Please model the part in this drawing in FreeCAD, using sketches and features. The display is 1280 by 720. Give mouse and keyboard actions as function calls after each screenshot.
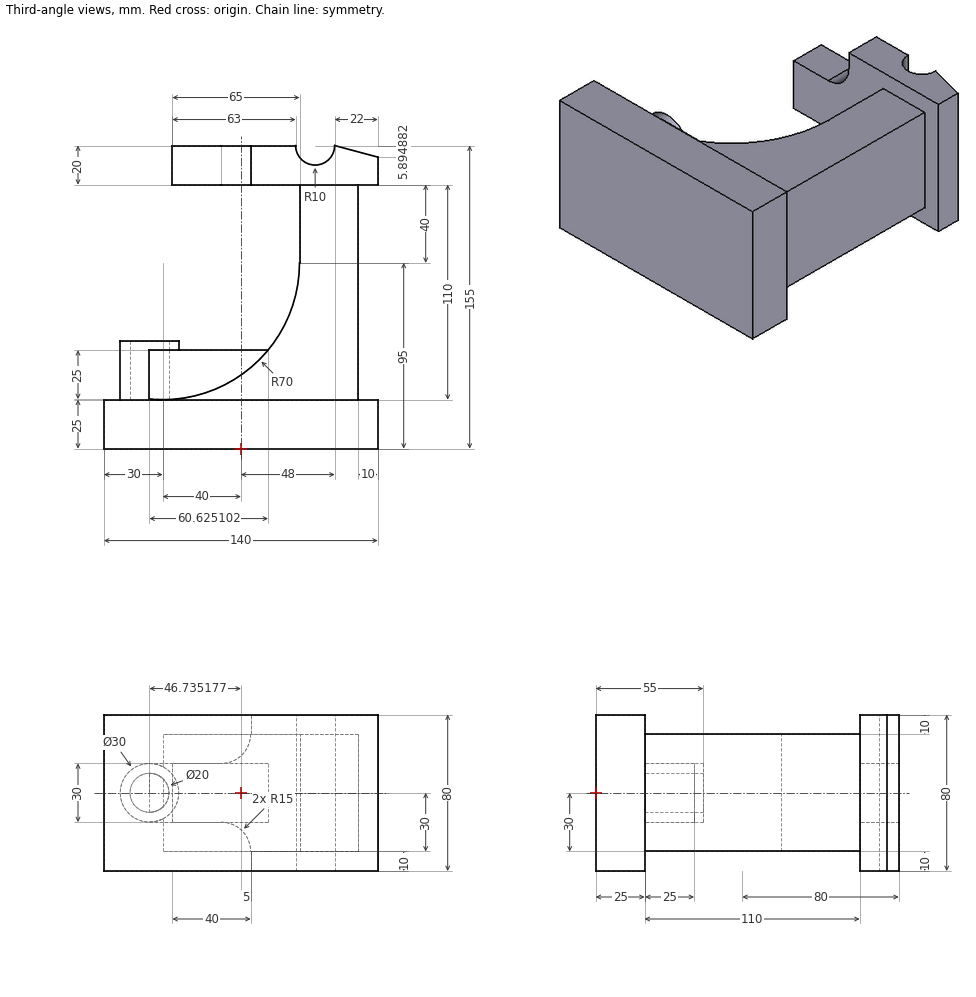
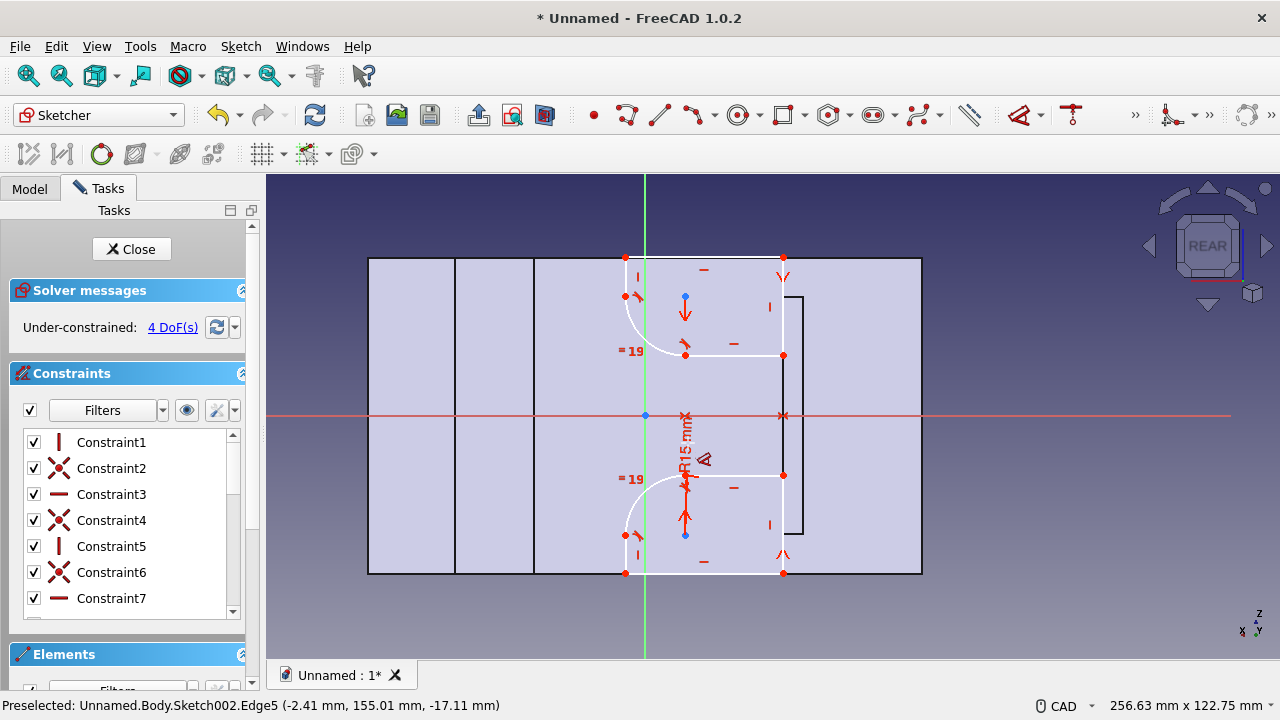
click(626, 547)
click(592, 554)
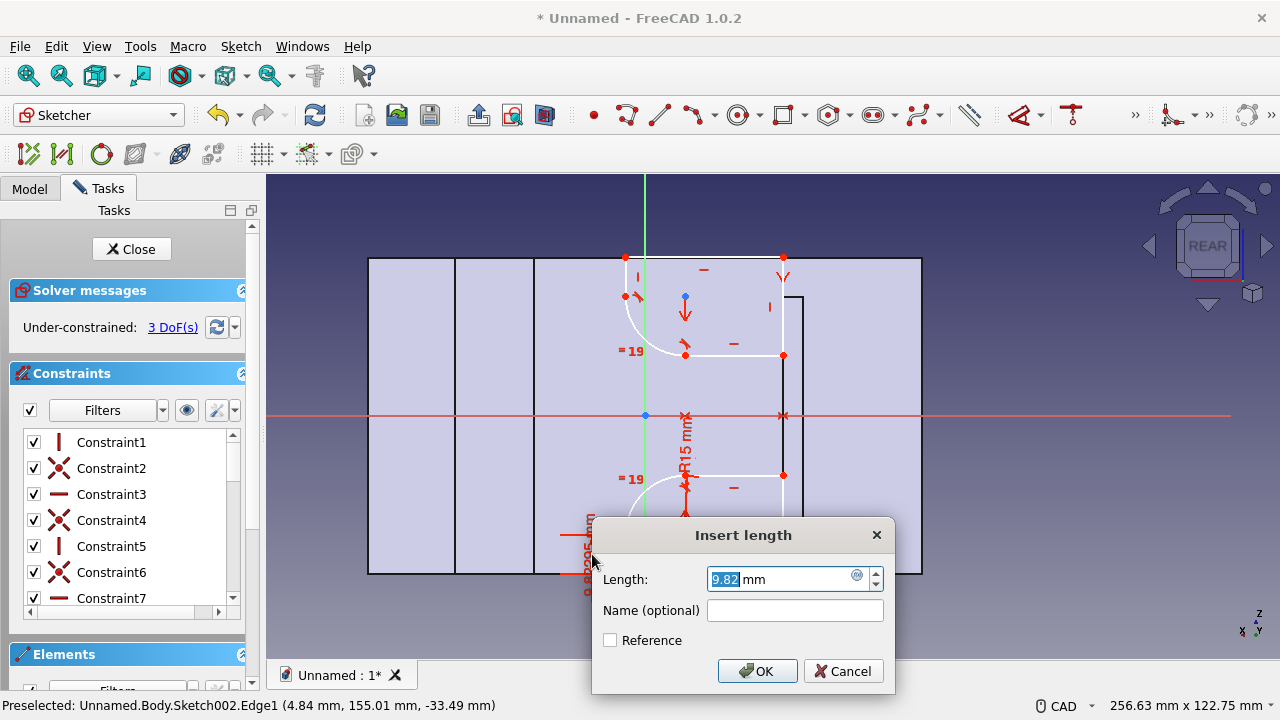
text(10)
key(Return)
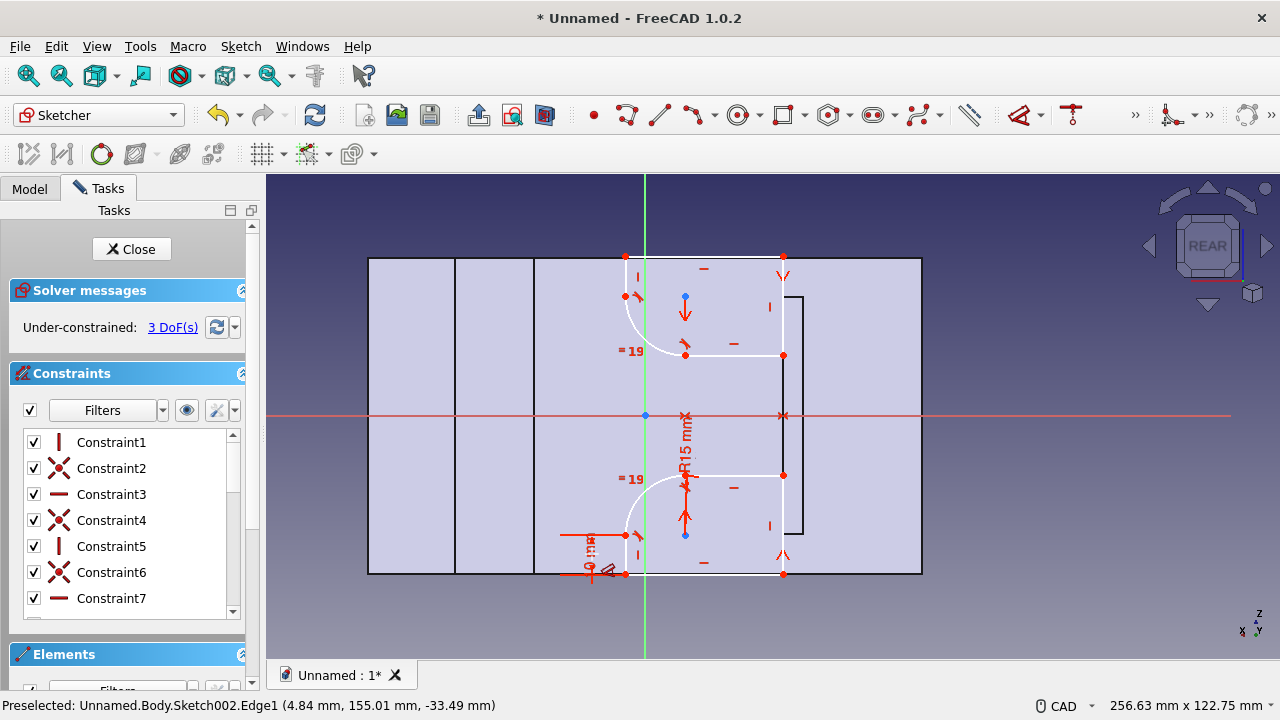
click(673, 575)
click(704, 609)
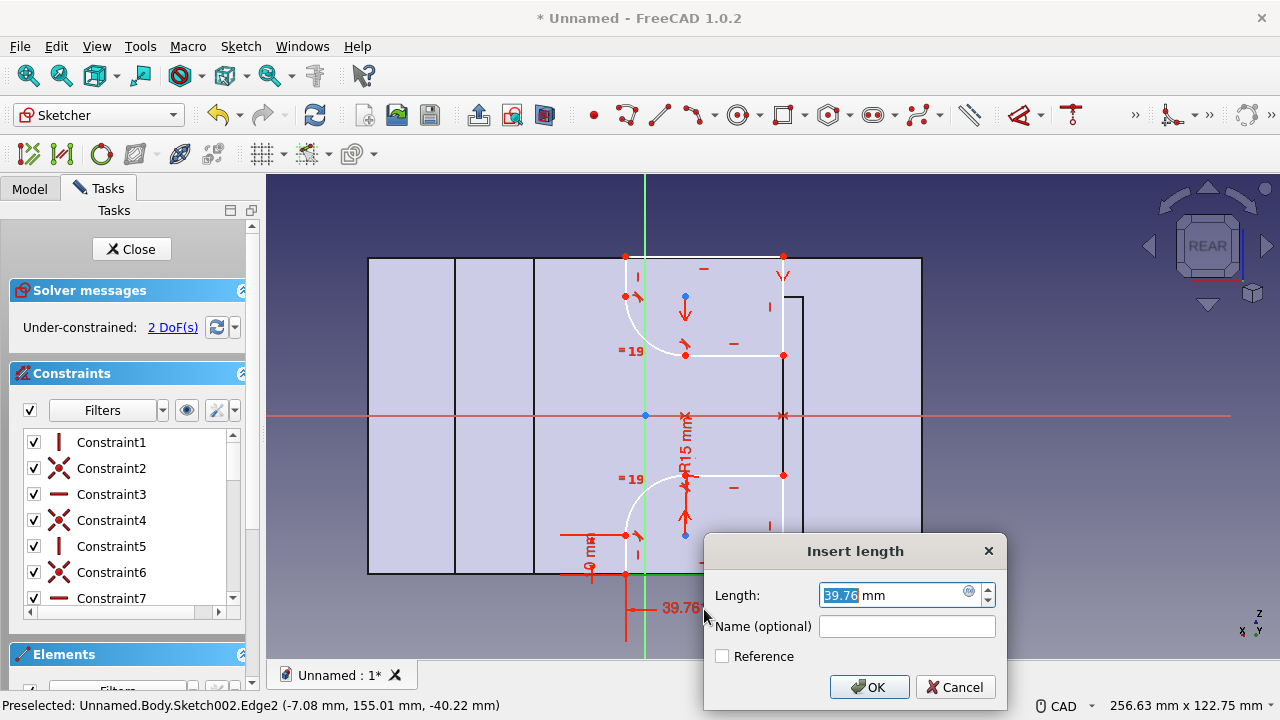
text(40)
key(Return)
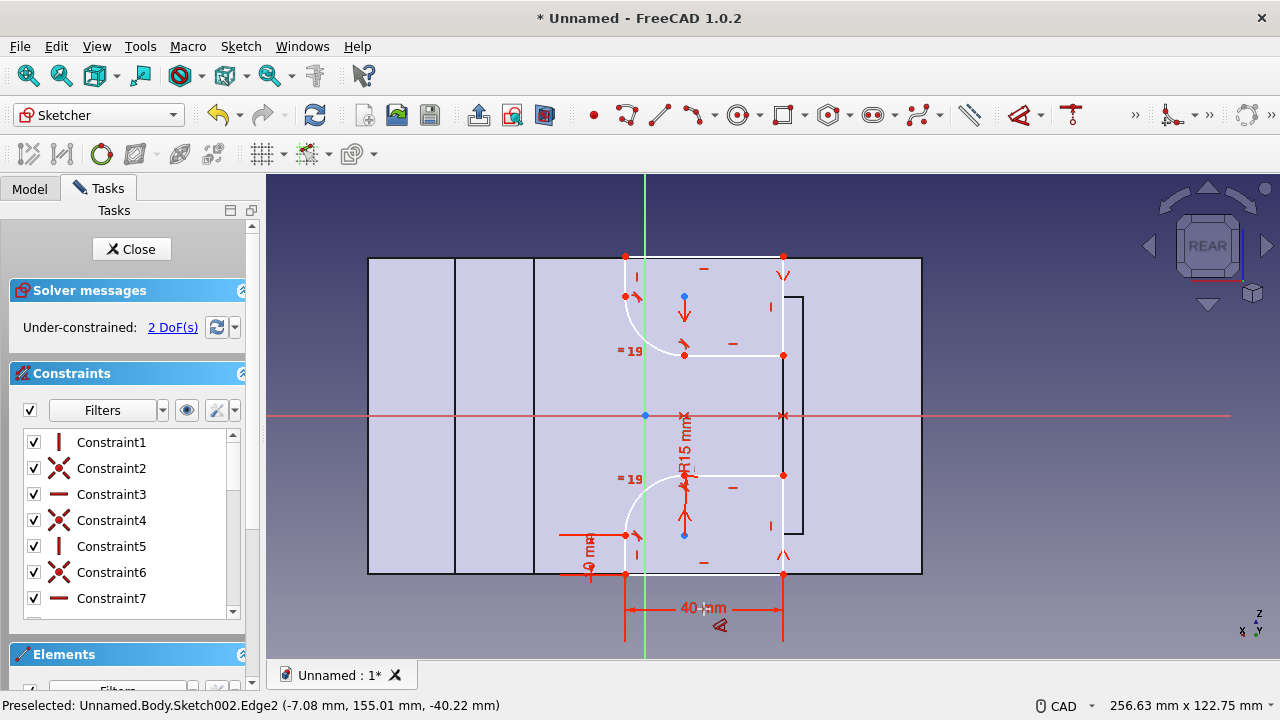
scroll(625, 535, up, 4)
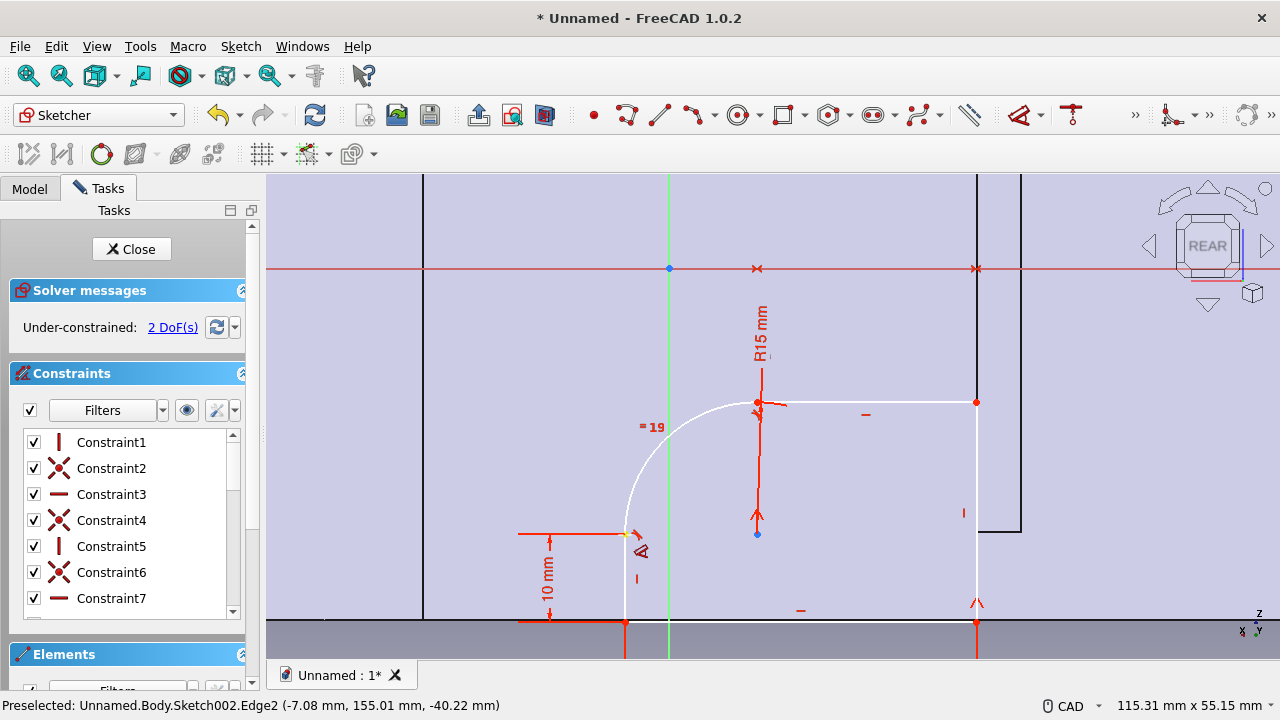
click(625, 534)
click(647, 568)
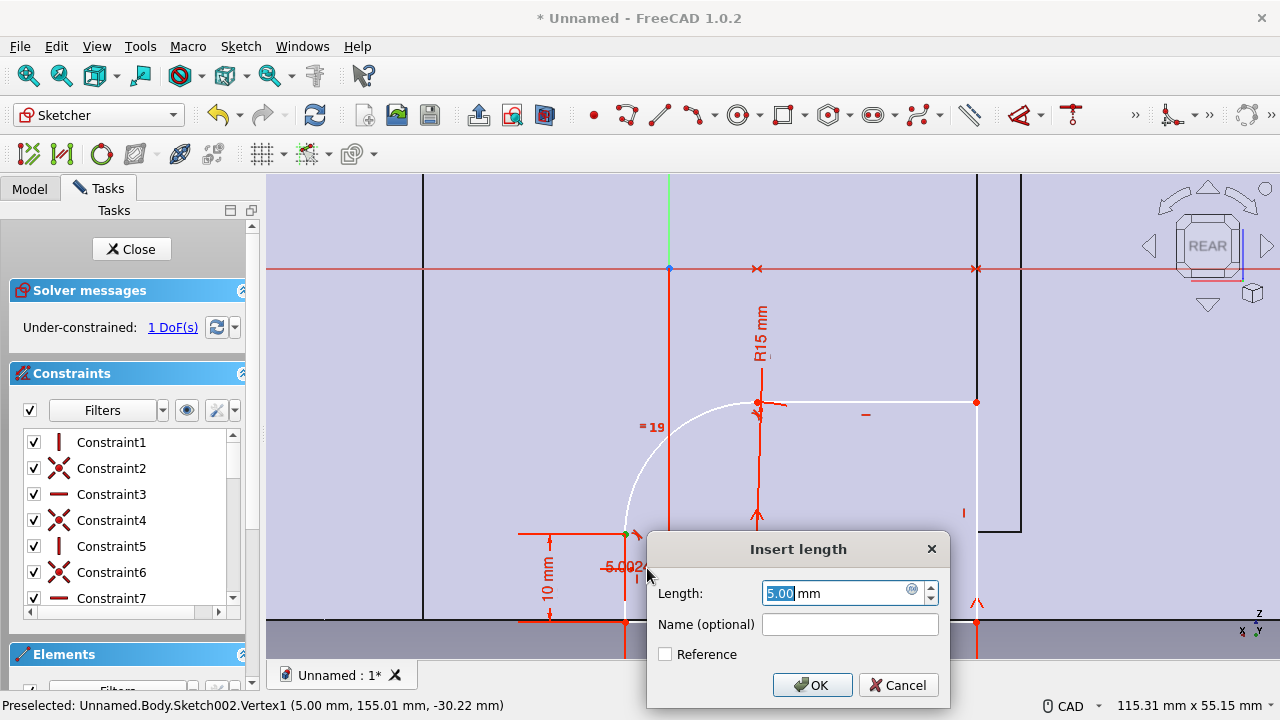
text(5)
key(Return)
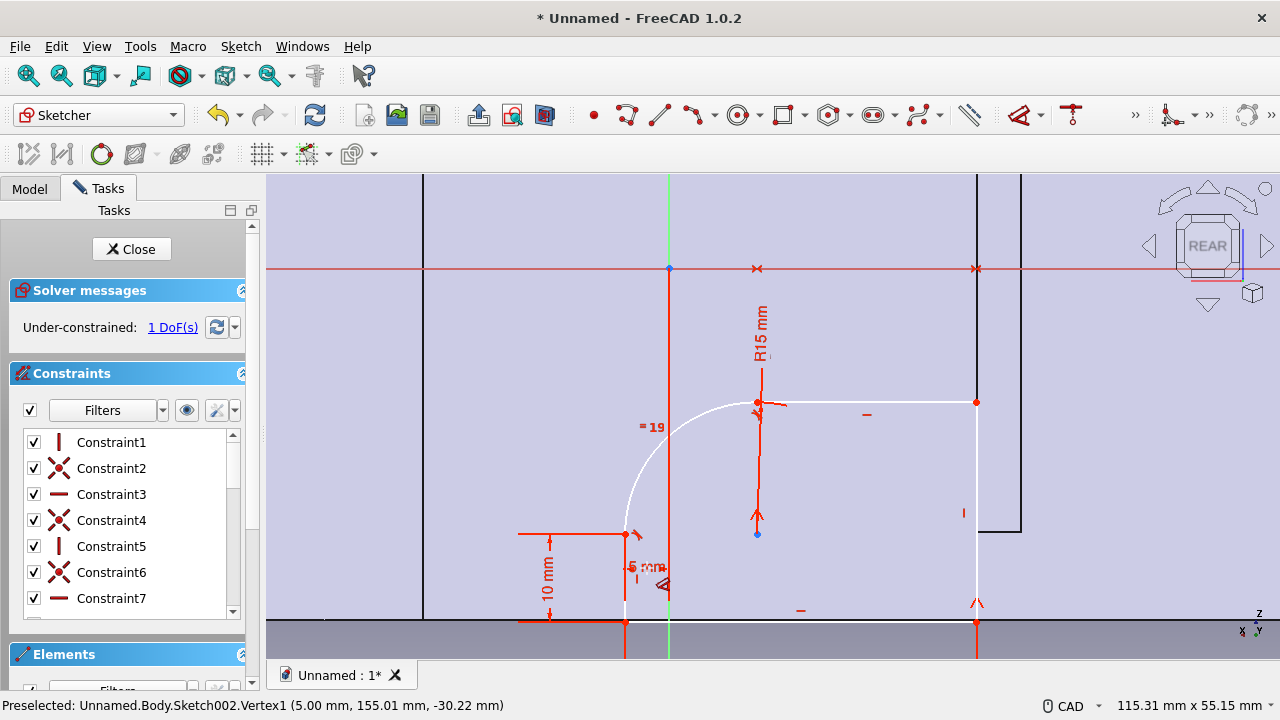
click(625, 534)
click(591, 401)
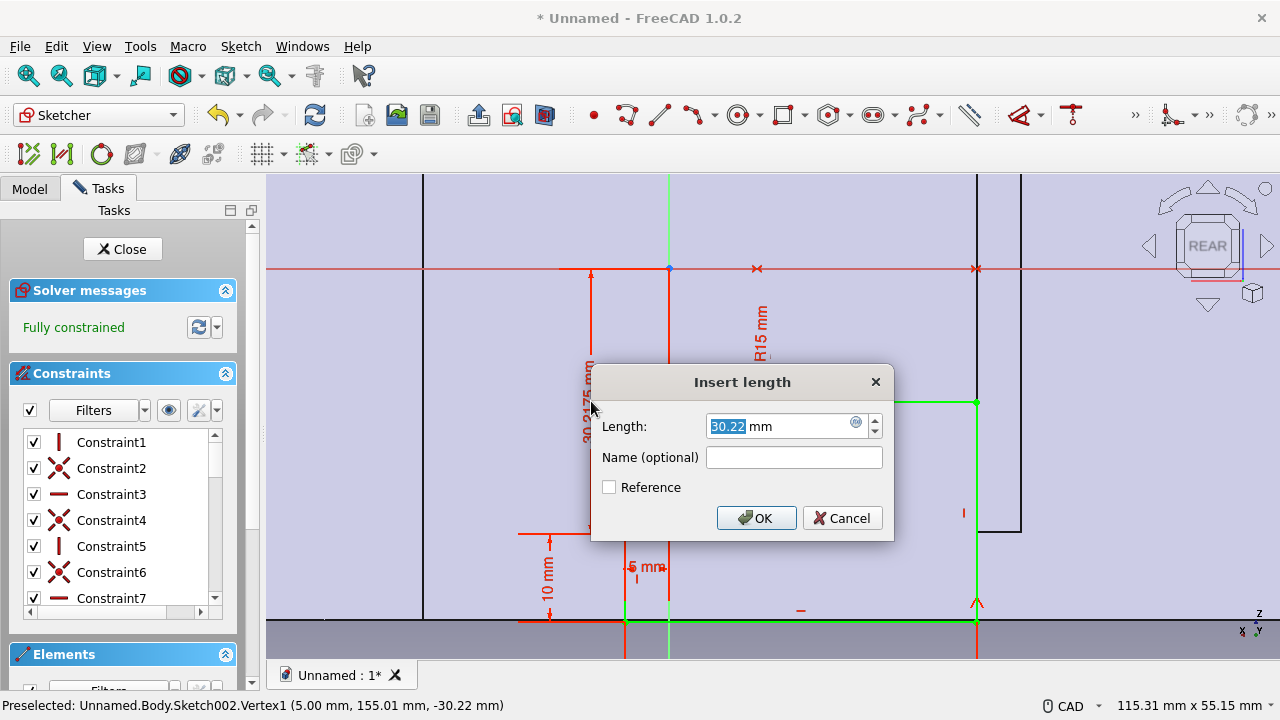
text(30)
key(Return)
key(Escape)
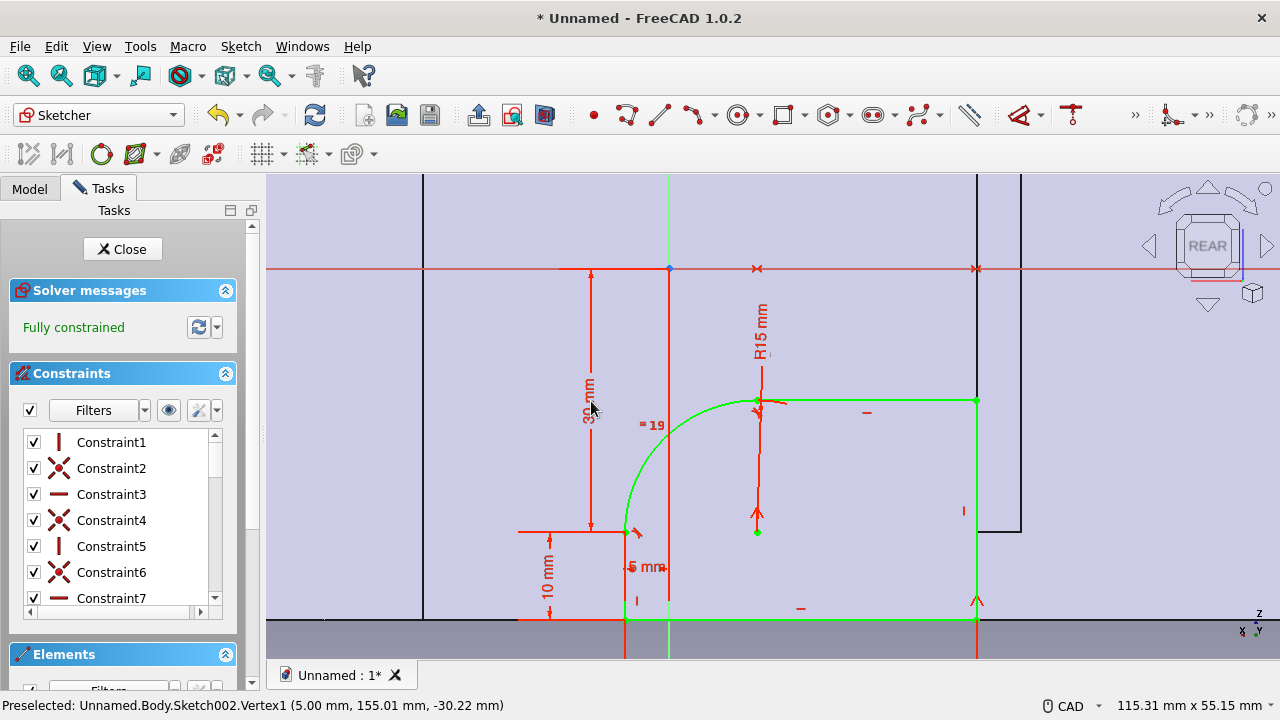
click(123, 249)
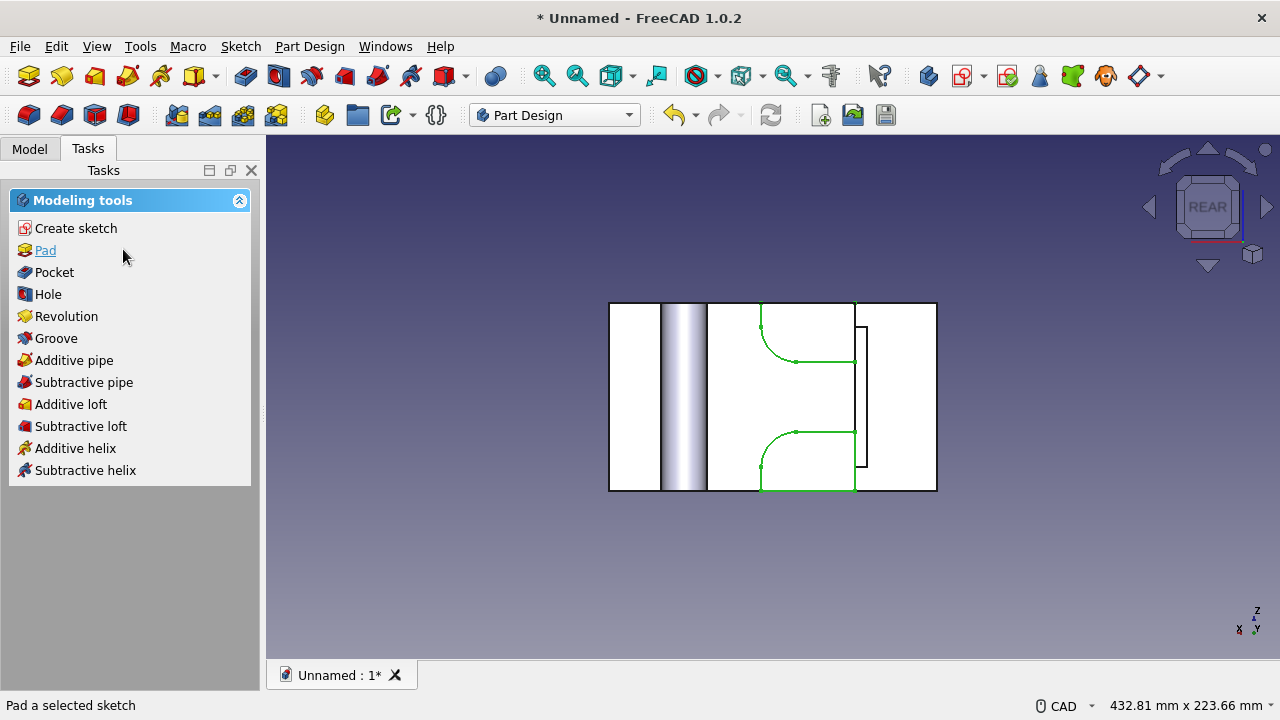
click(246, 76)